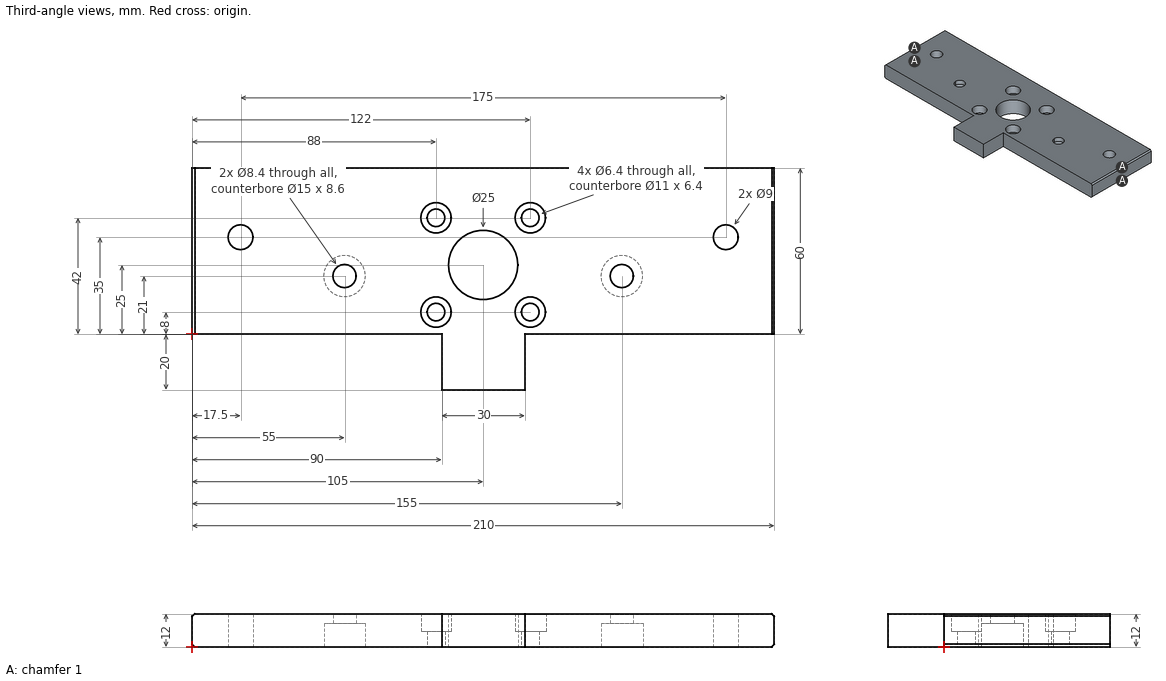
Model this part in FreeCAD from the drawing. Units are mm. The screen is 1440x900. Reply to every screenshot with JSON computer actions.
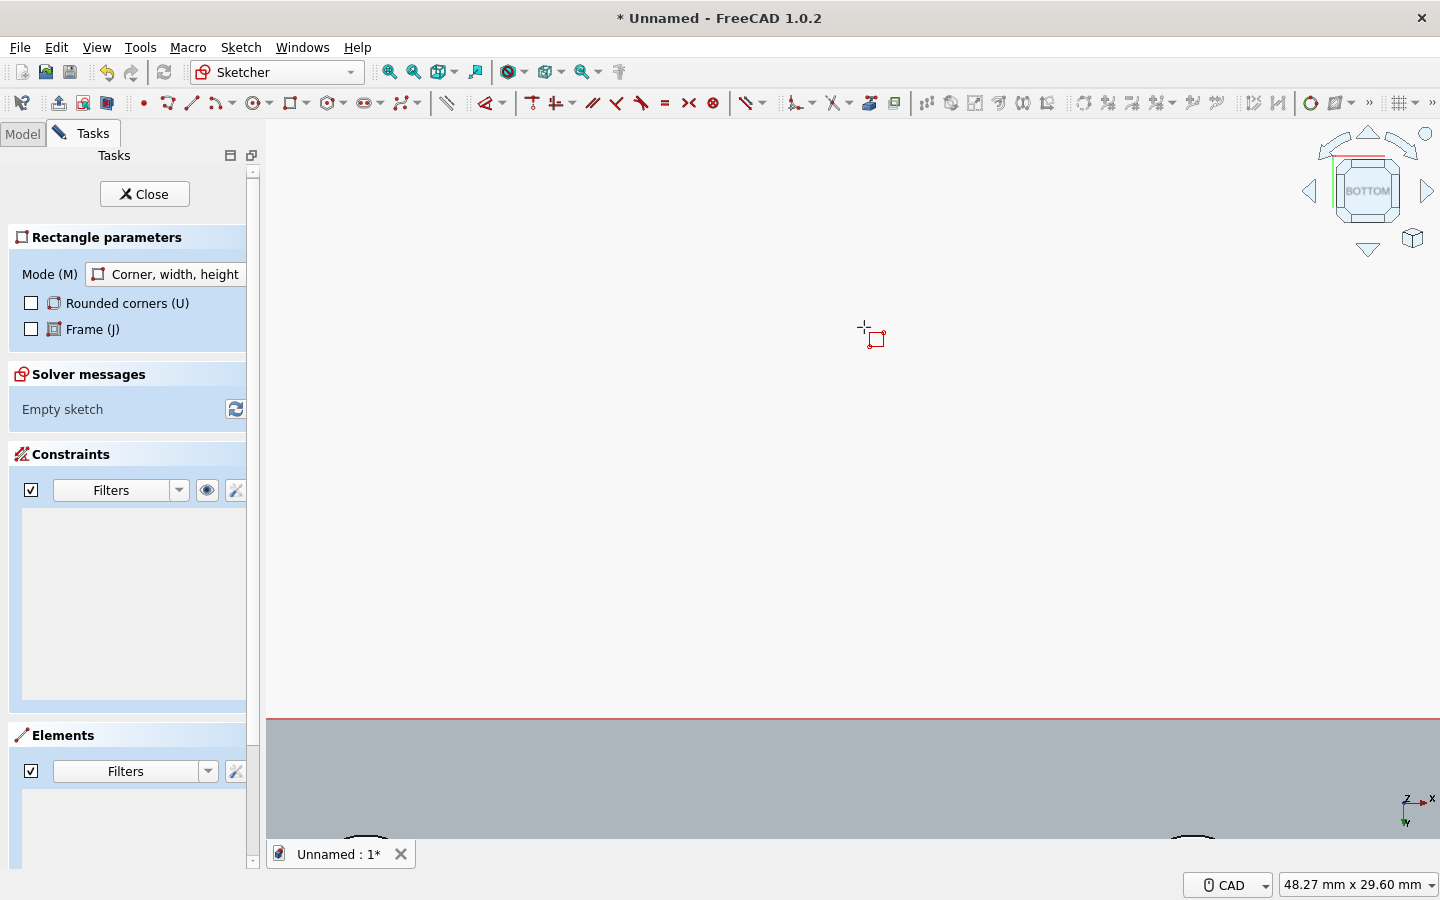
{"action": "left_click", "coordinate": [415, 232]}
{"action": "left_click", "coordinate": [1144, 719]}
{"action": "key", "text": "Escape"}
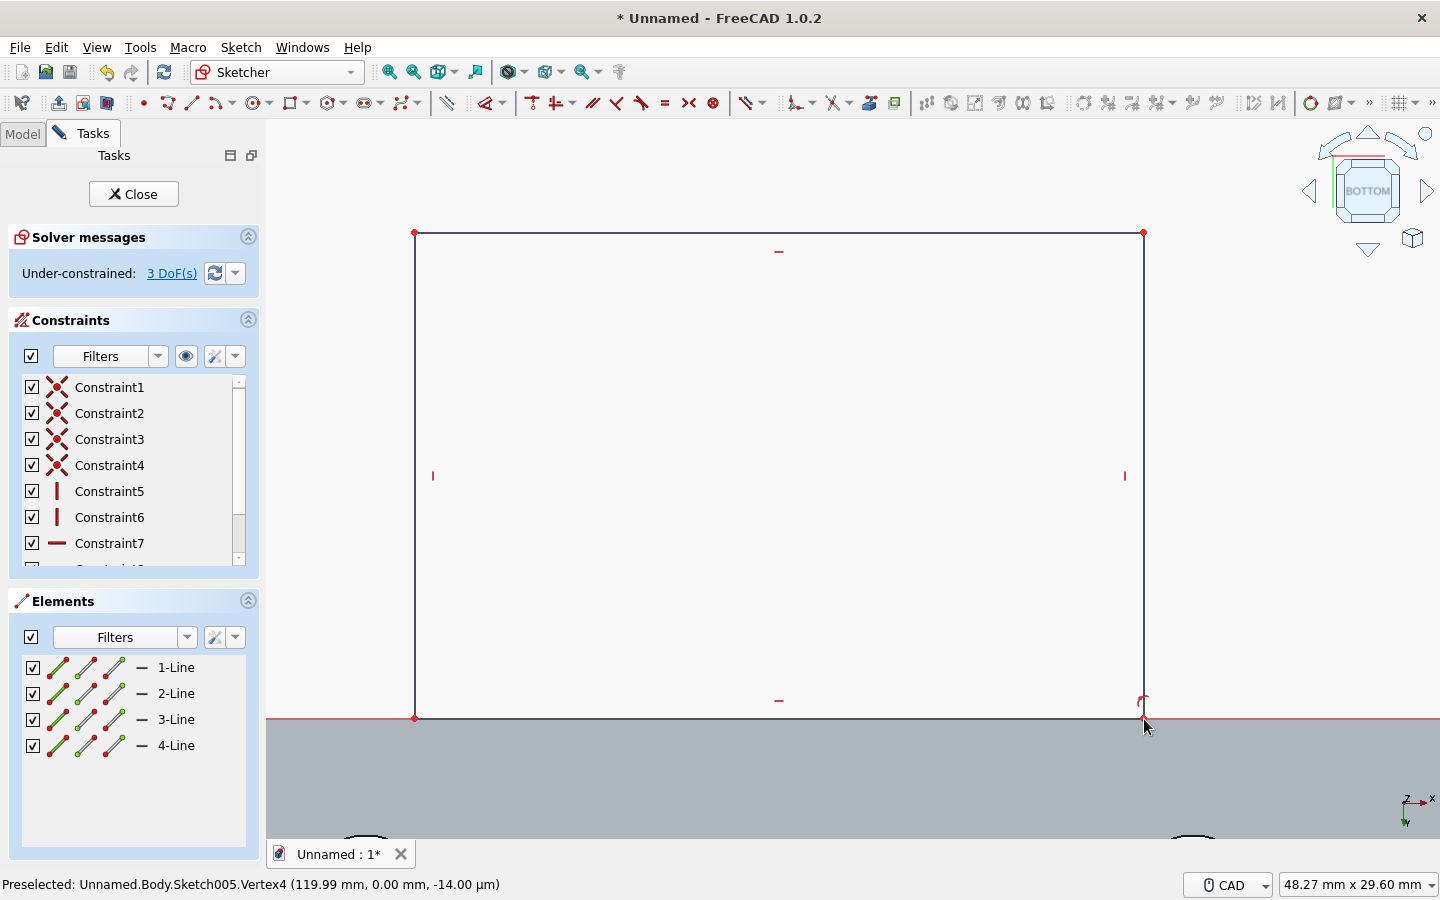
{"action": "left_click", "coordinate": [486, 104]}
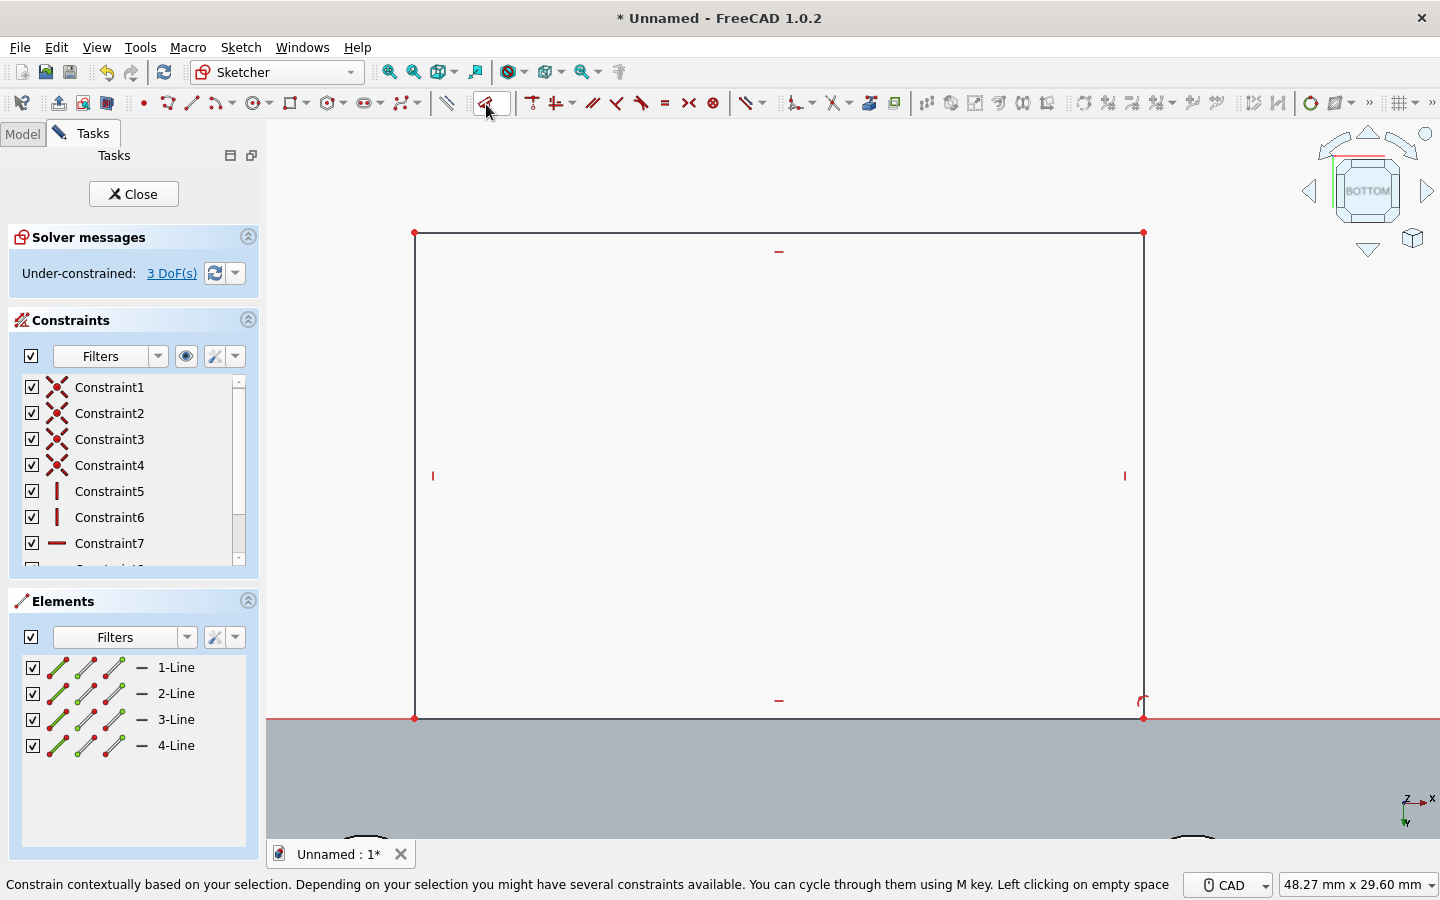
{"action": "left_click", "coordinate": [415, 379]}
{"action": "left_click", "coordinate": [381, 476]}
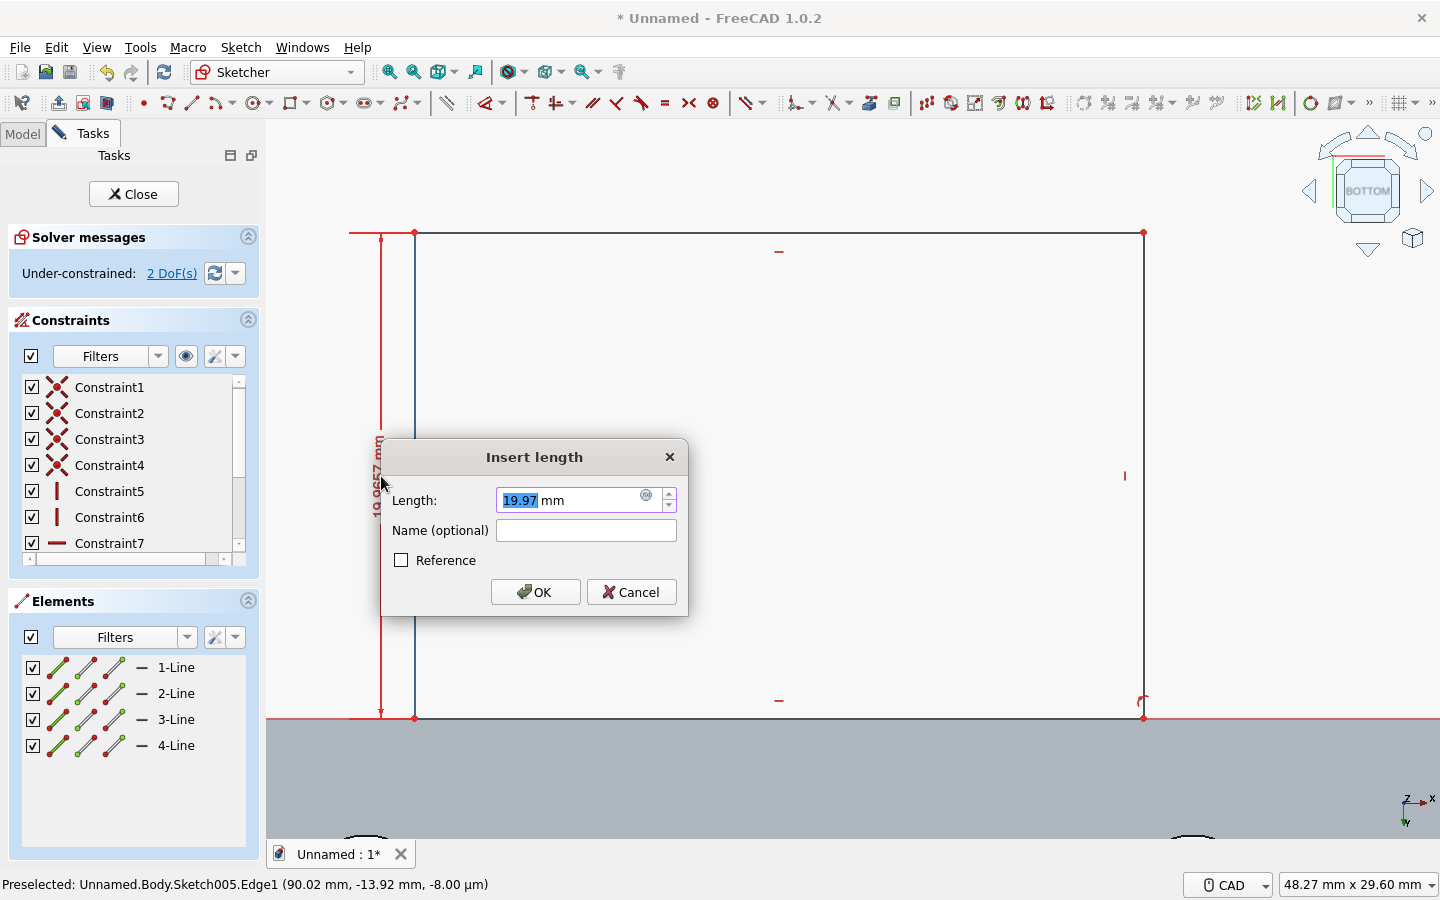
{"action": "type", "text": "20"}
{"action": "key", "text": "Return"}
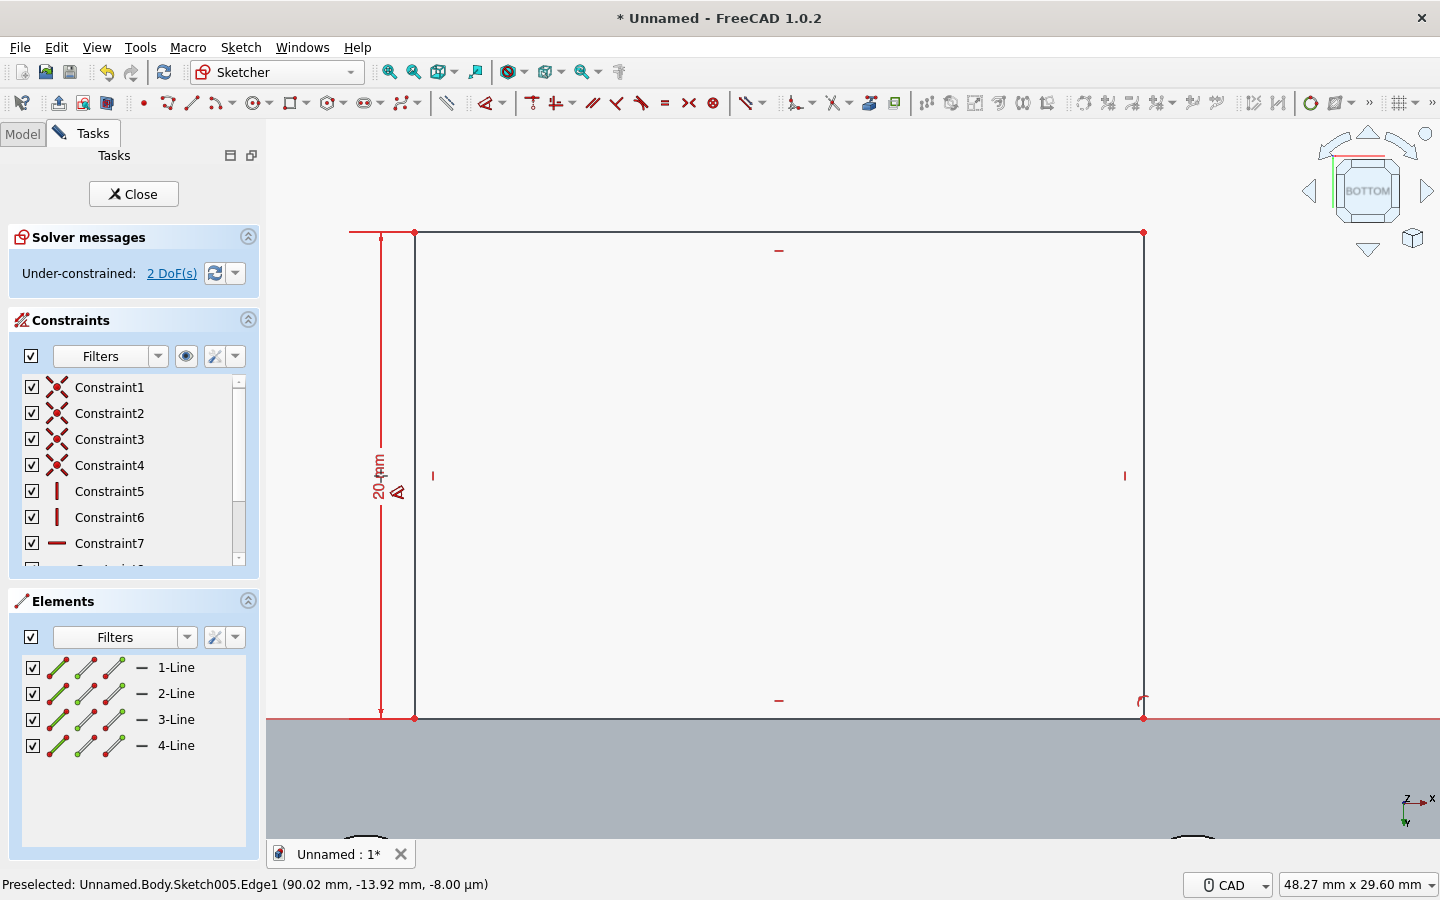
{"action": "left_click", "coordinate": [634, 719]}
{"action": "left_click", "coordinate": [779, 753]}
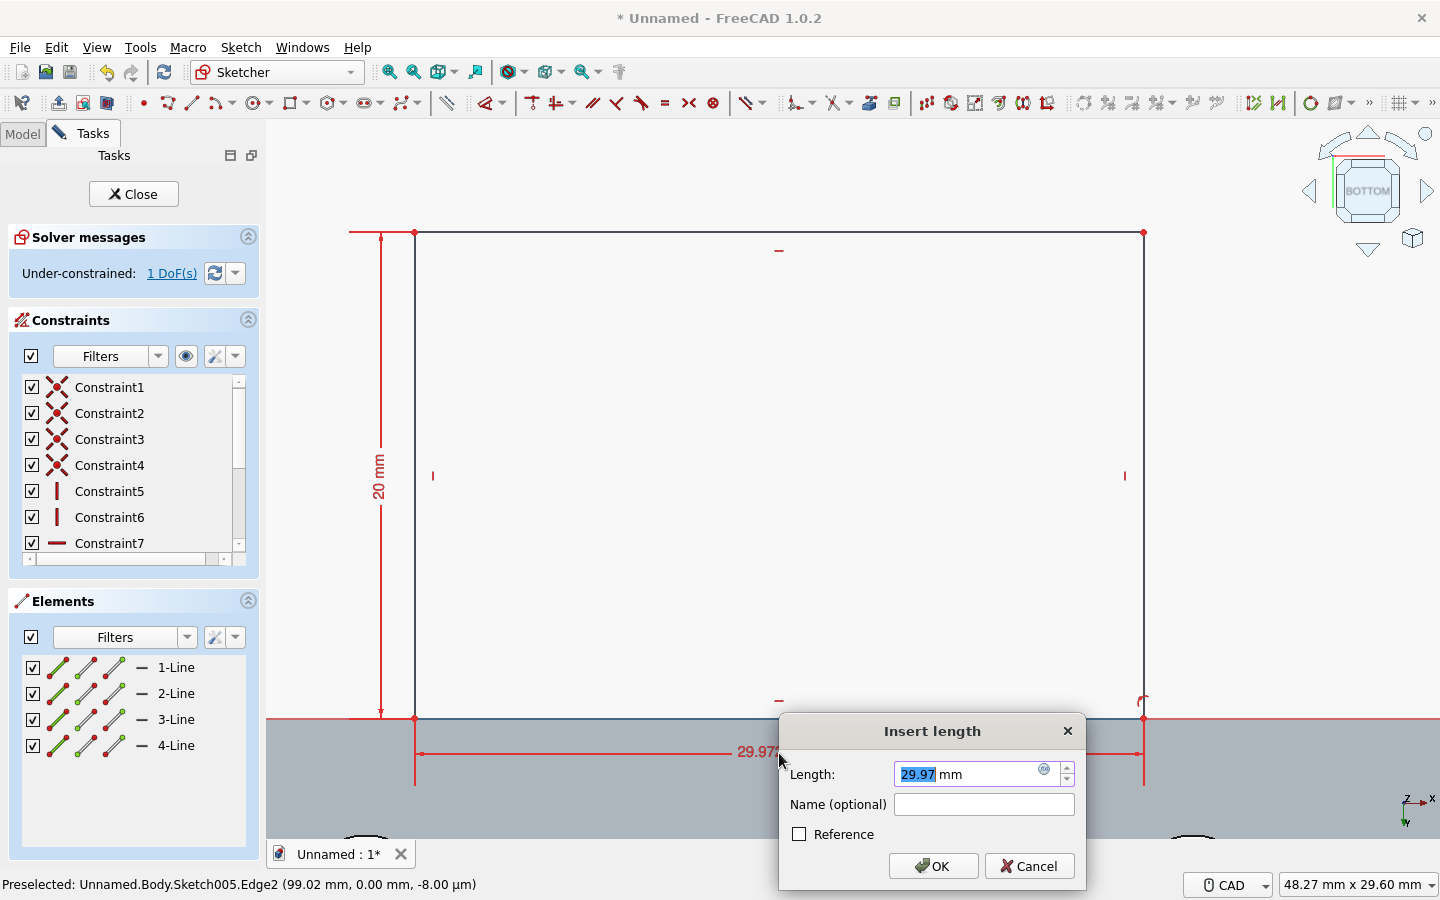
{"action": "type", "text": "30"}
{"action": "key", "text": "Return"}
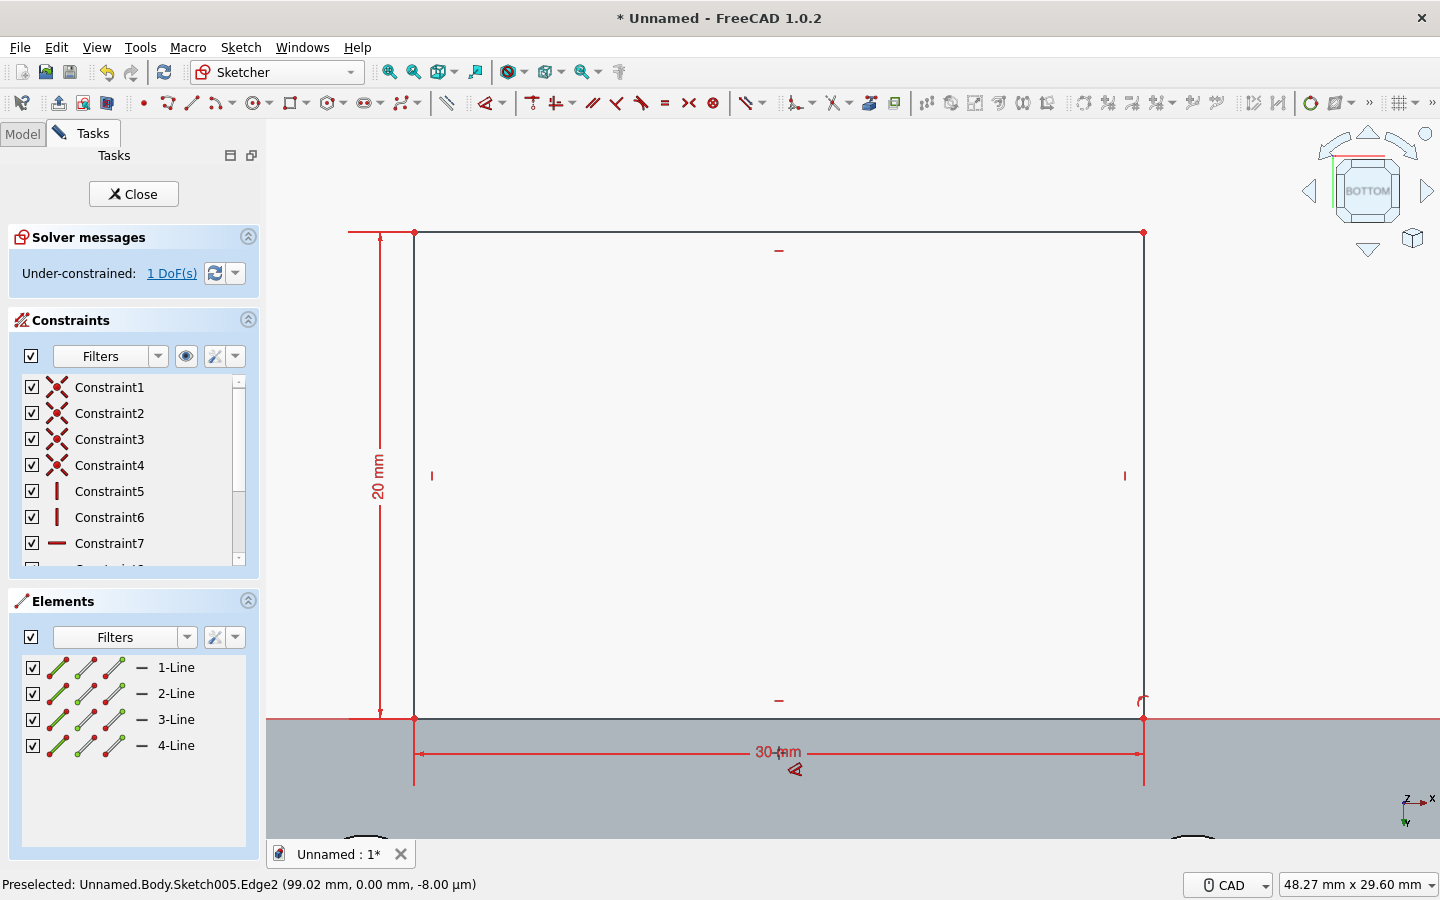
{"action": "left_click", "coordinate": [414, 232]}
{"action": "left_click", "coordinate": [354, 753]}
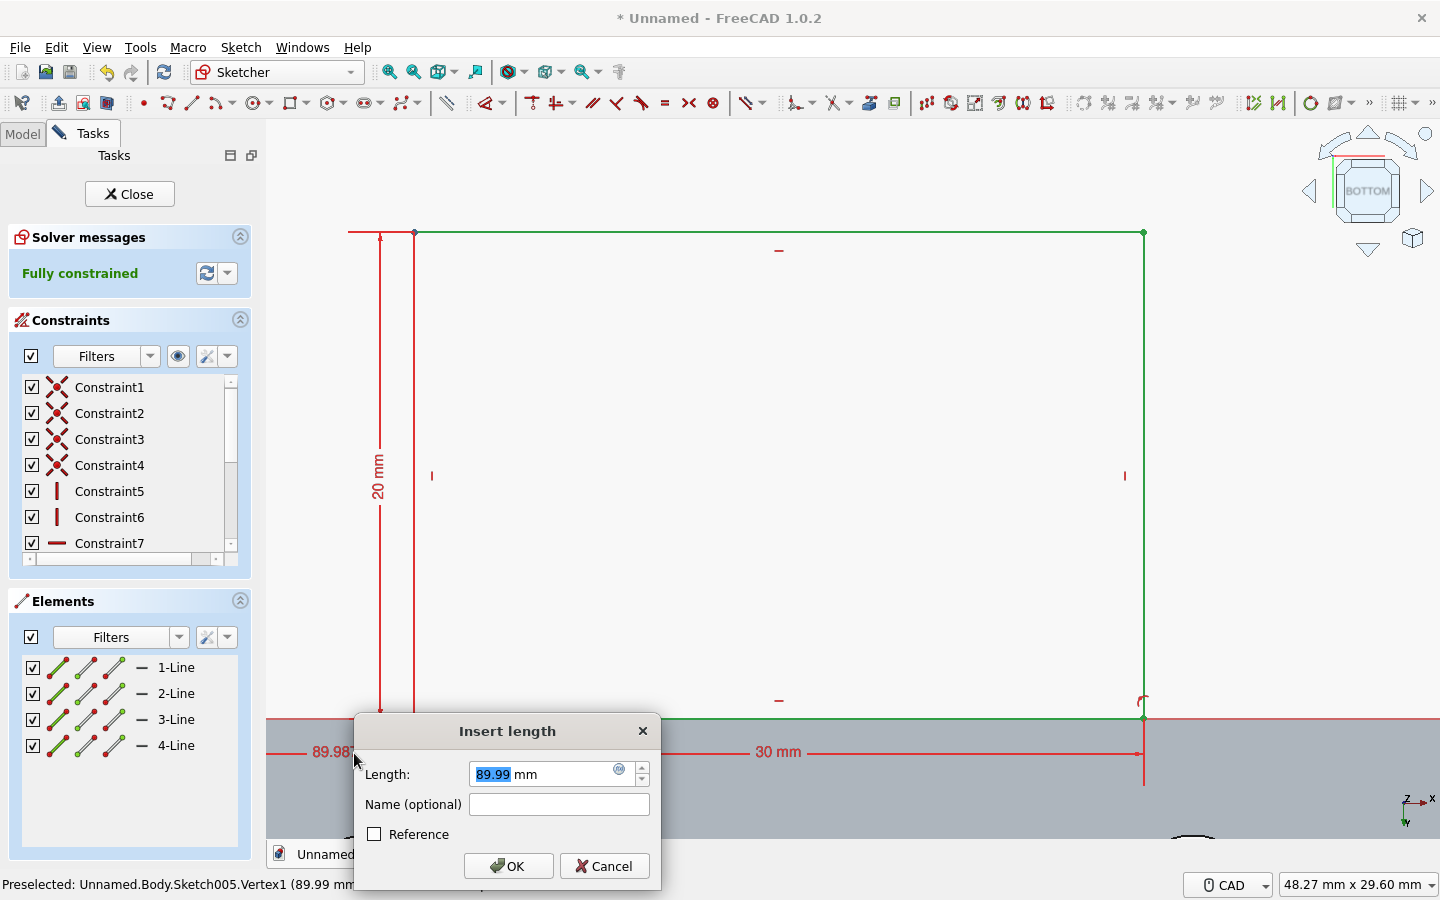
{"action": "type", "text": "90"}
{"action": "key", "text": "Return"}
{"action": "key", "text": "Escape"}